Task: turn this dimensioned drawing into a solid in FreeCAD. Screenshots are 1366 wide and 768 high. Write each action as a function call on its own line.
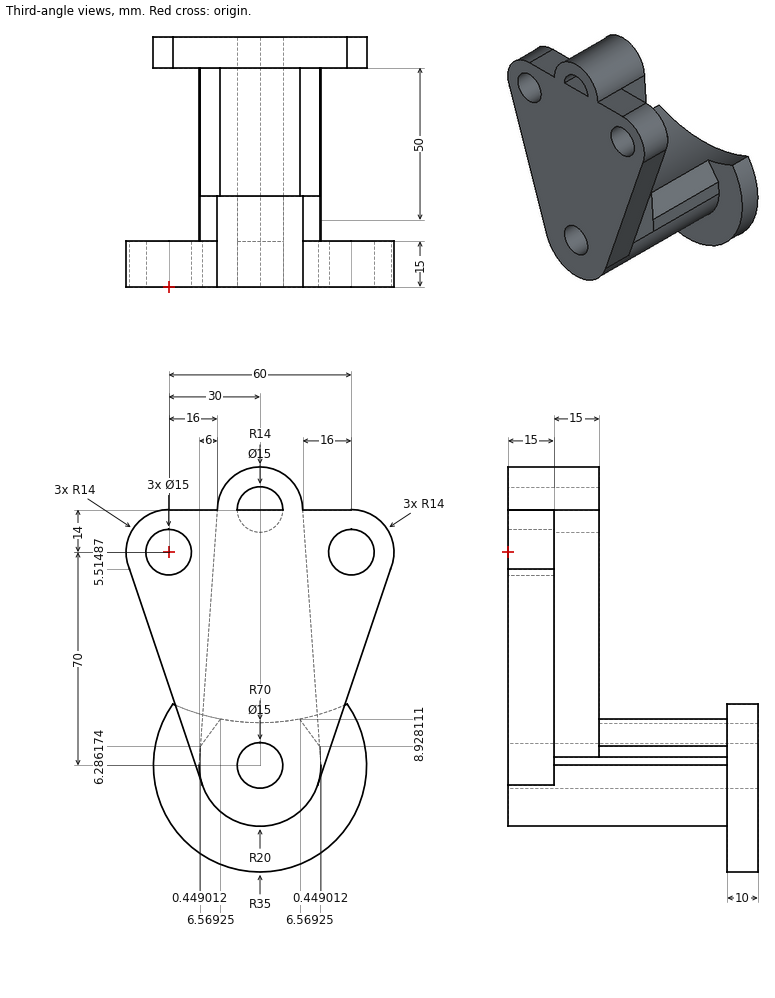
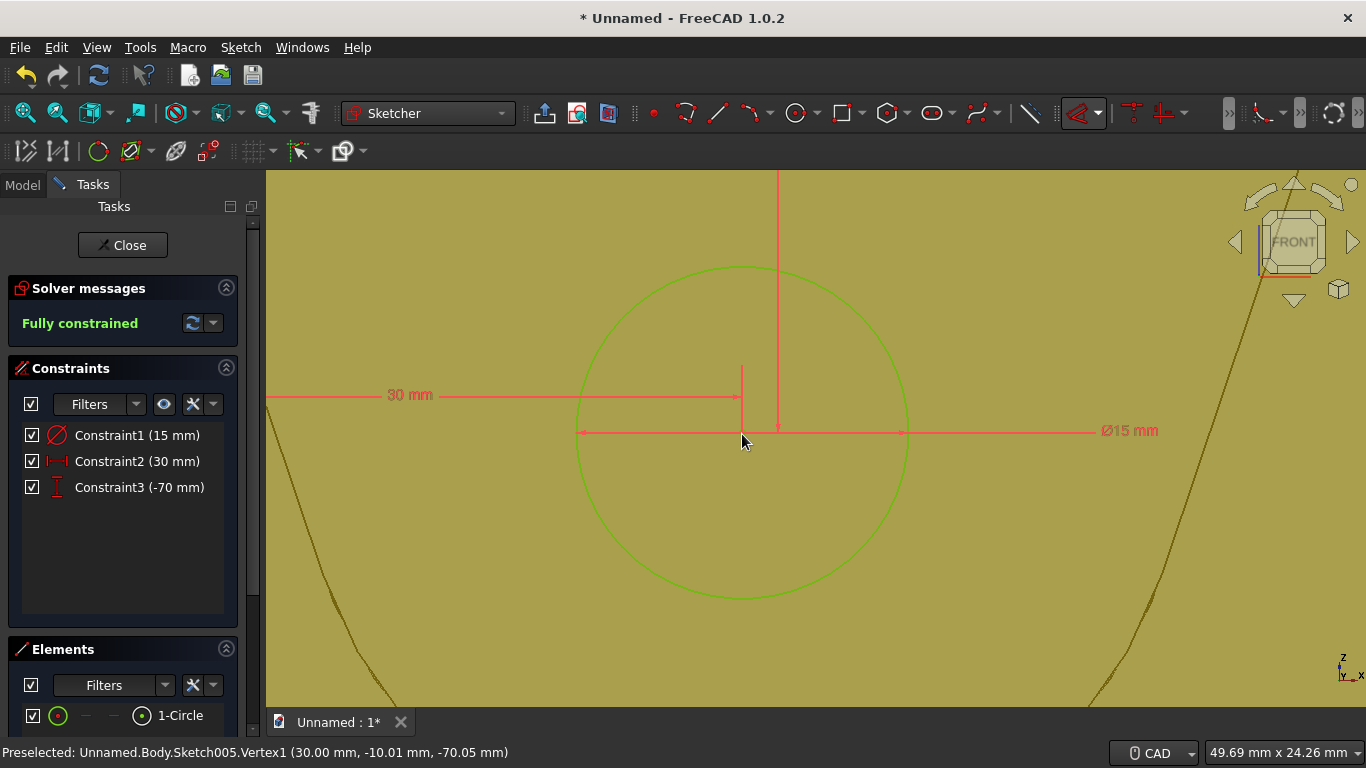
click(123, 245)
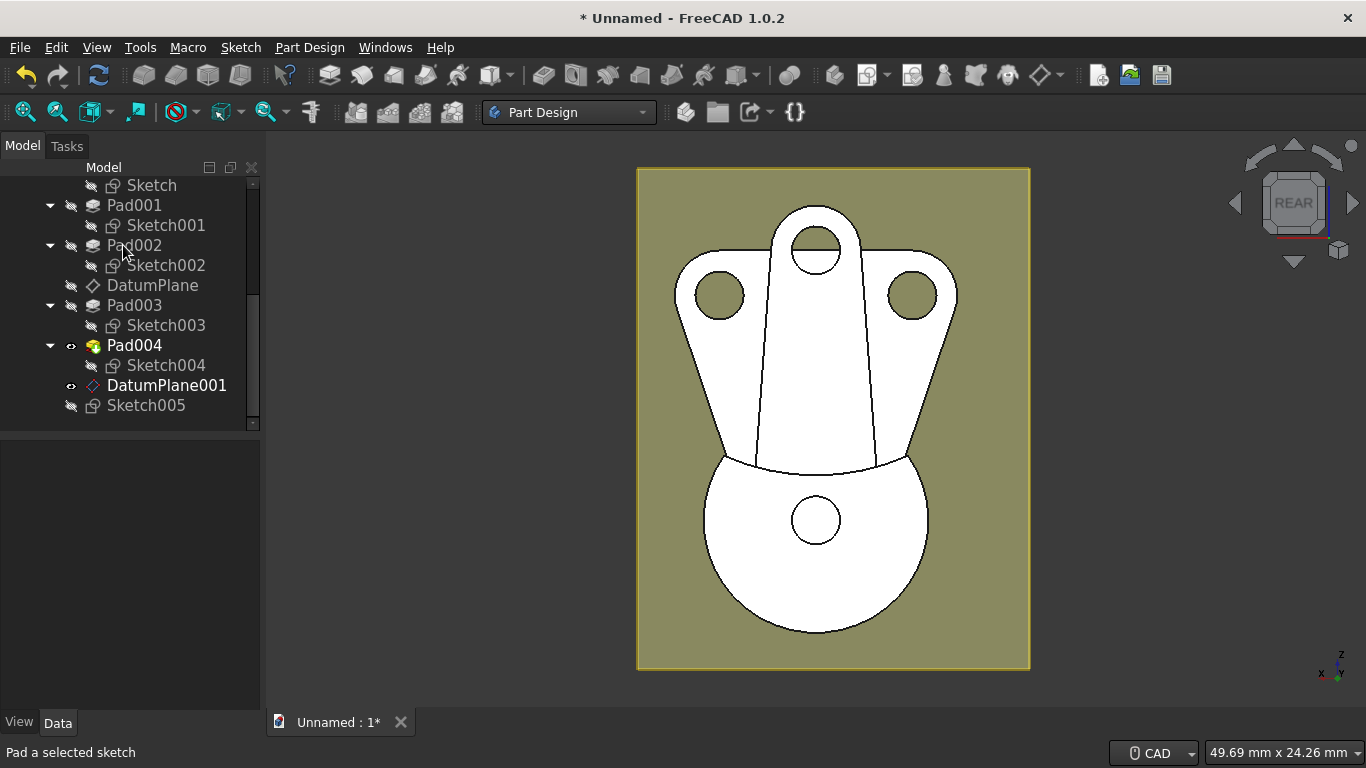
click(544, 76)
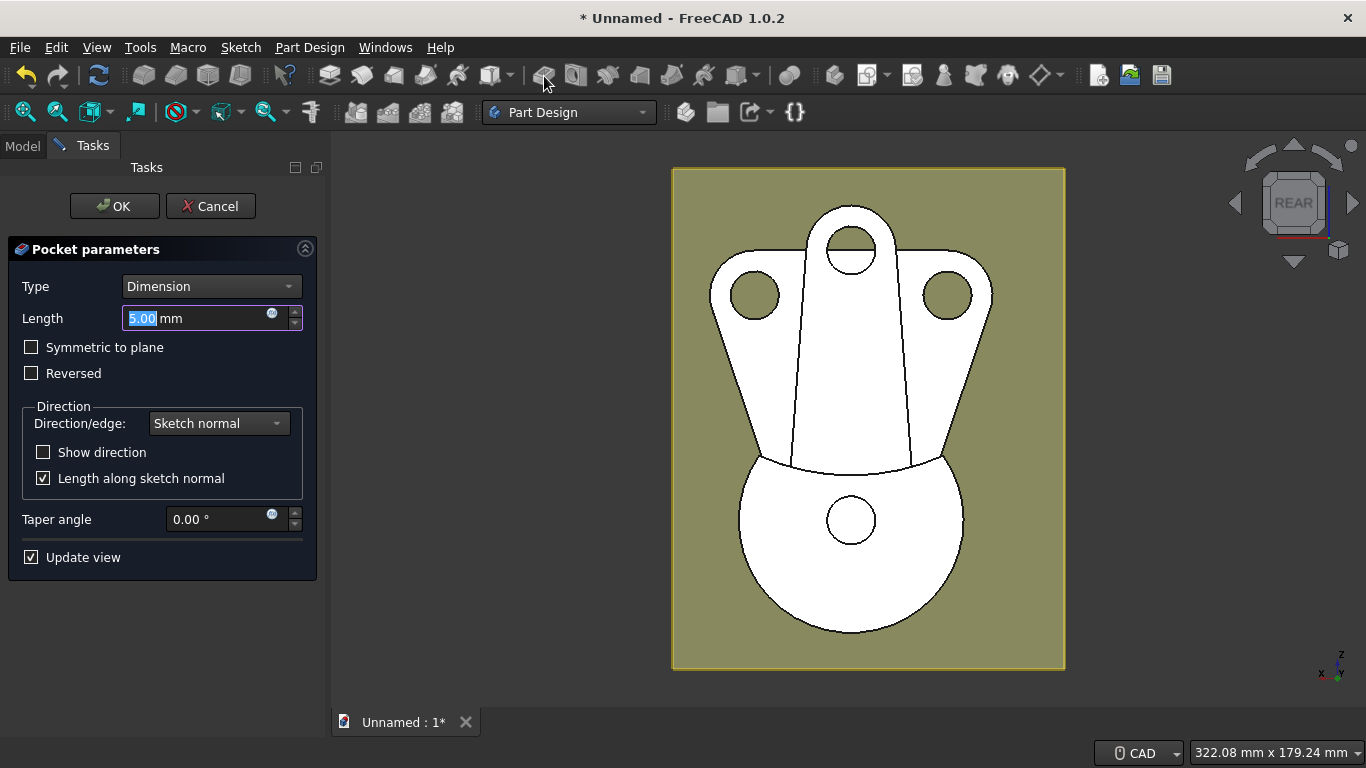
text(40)
key(Tab)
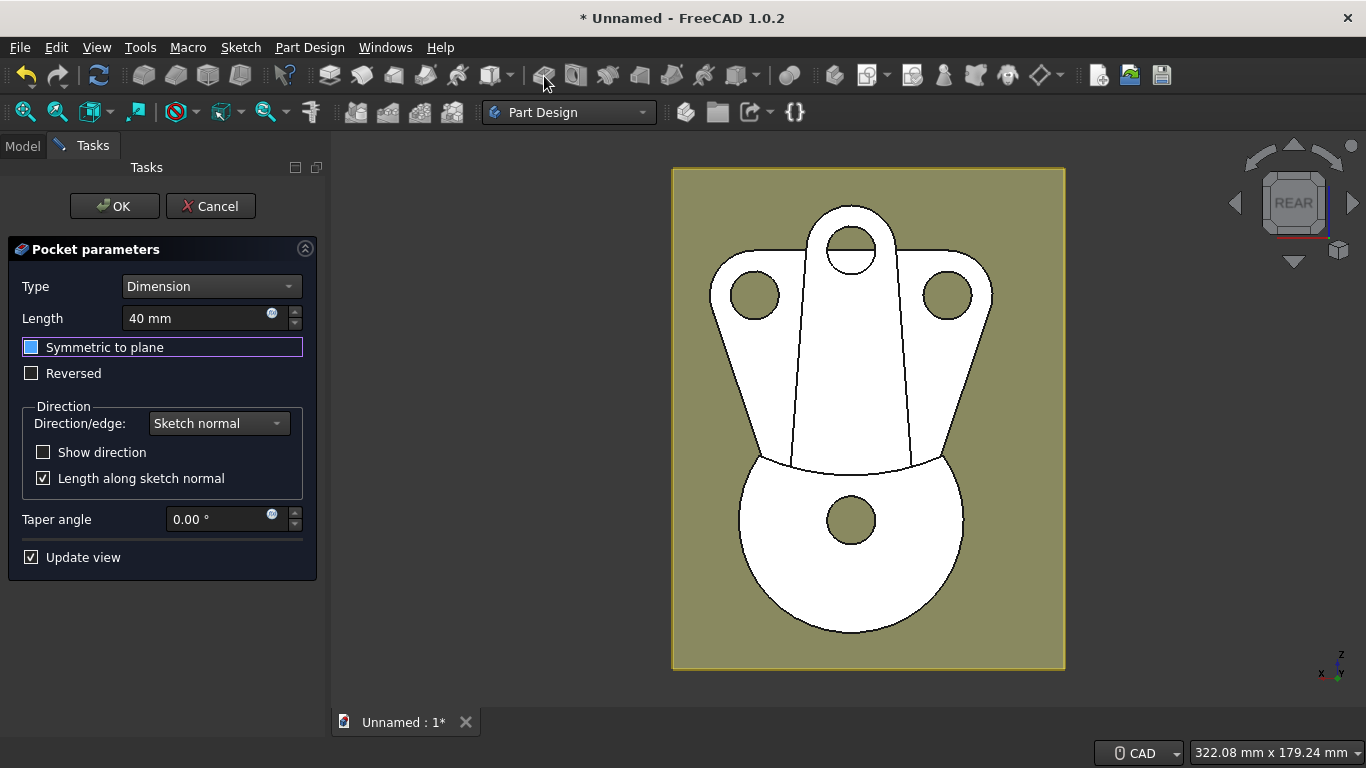
click(115, 206)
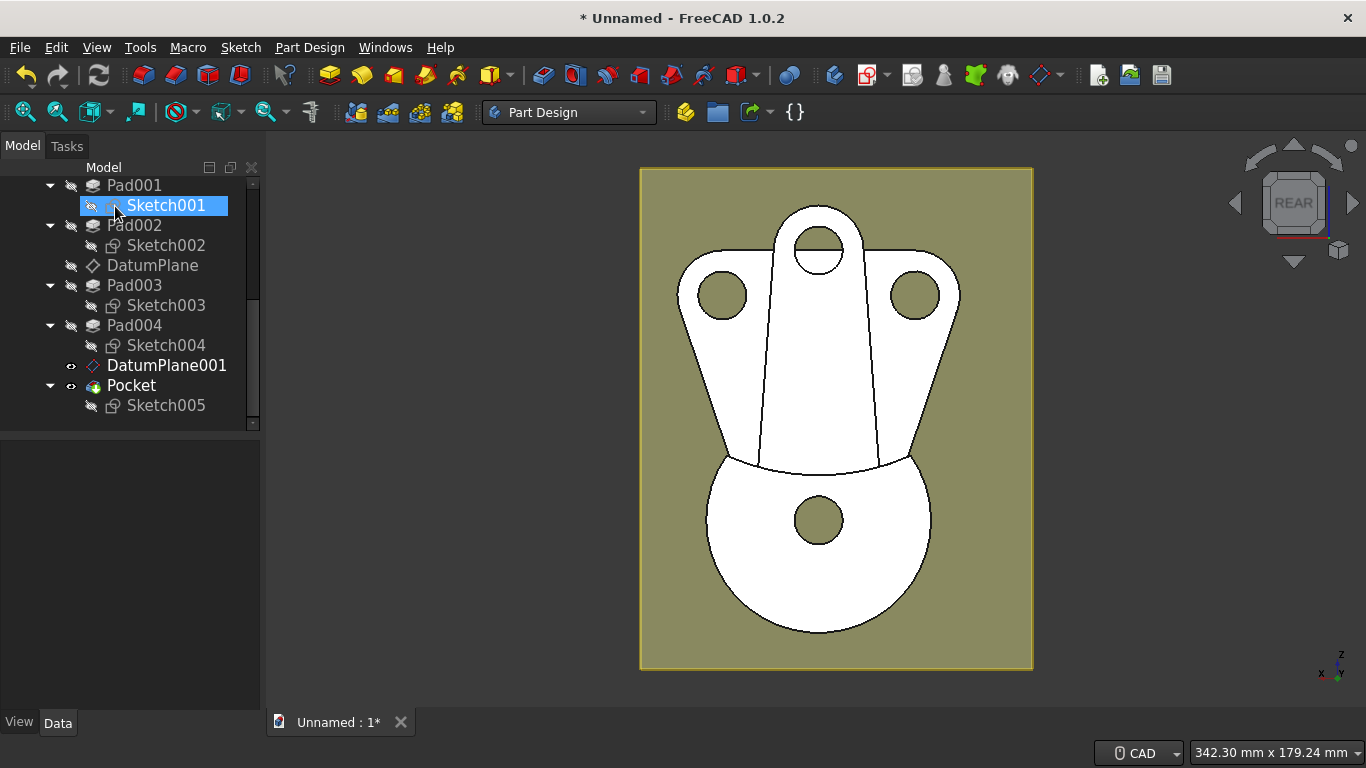
click(116, 366)
key(space)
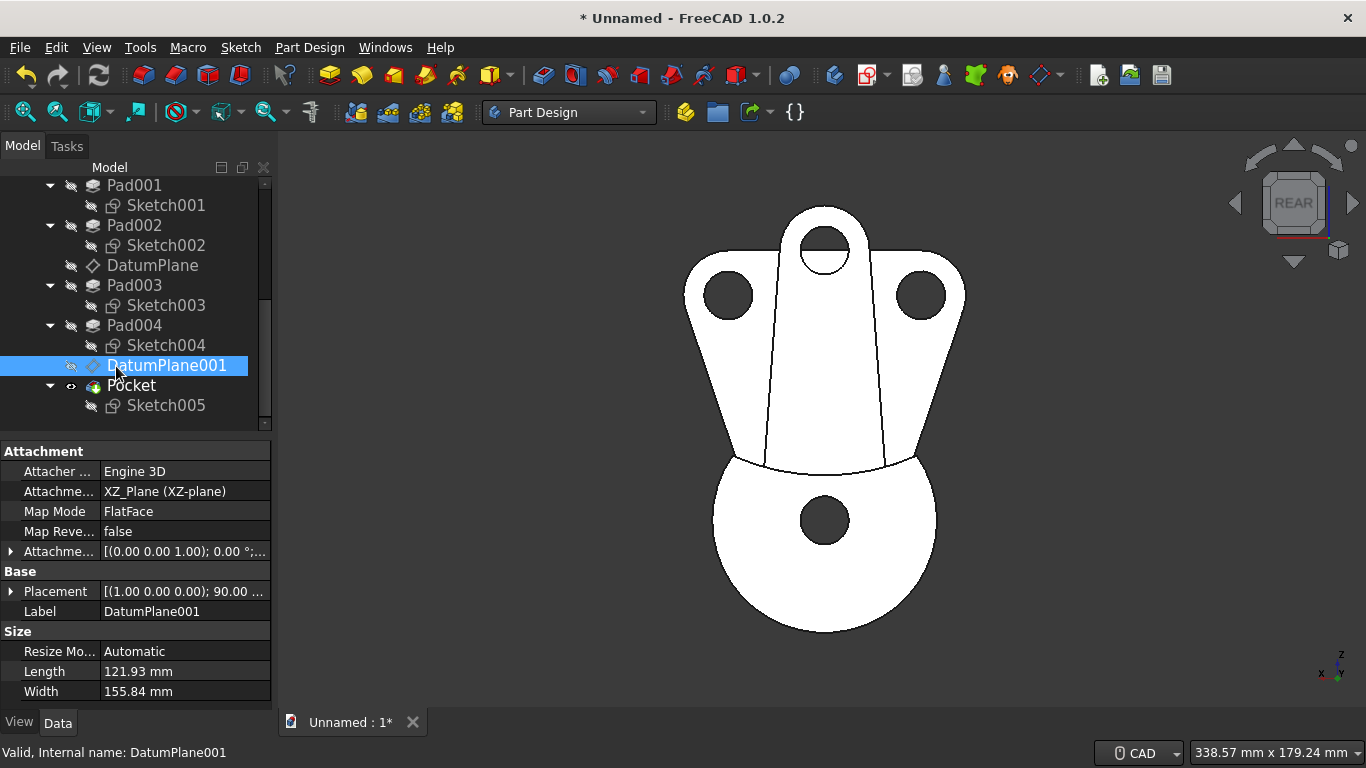
key(0)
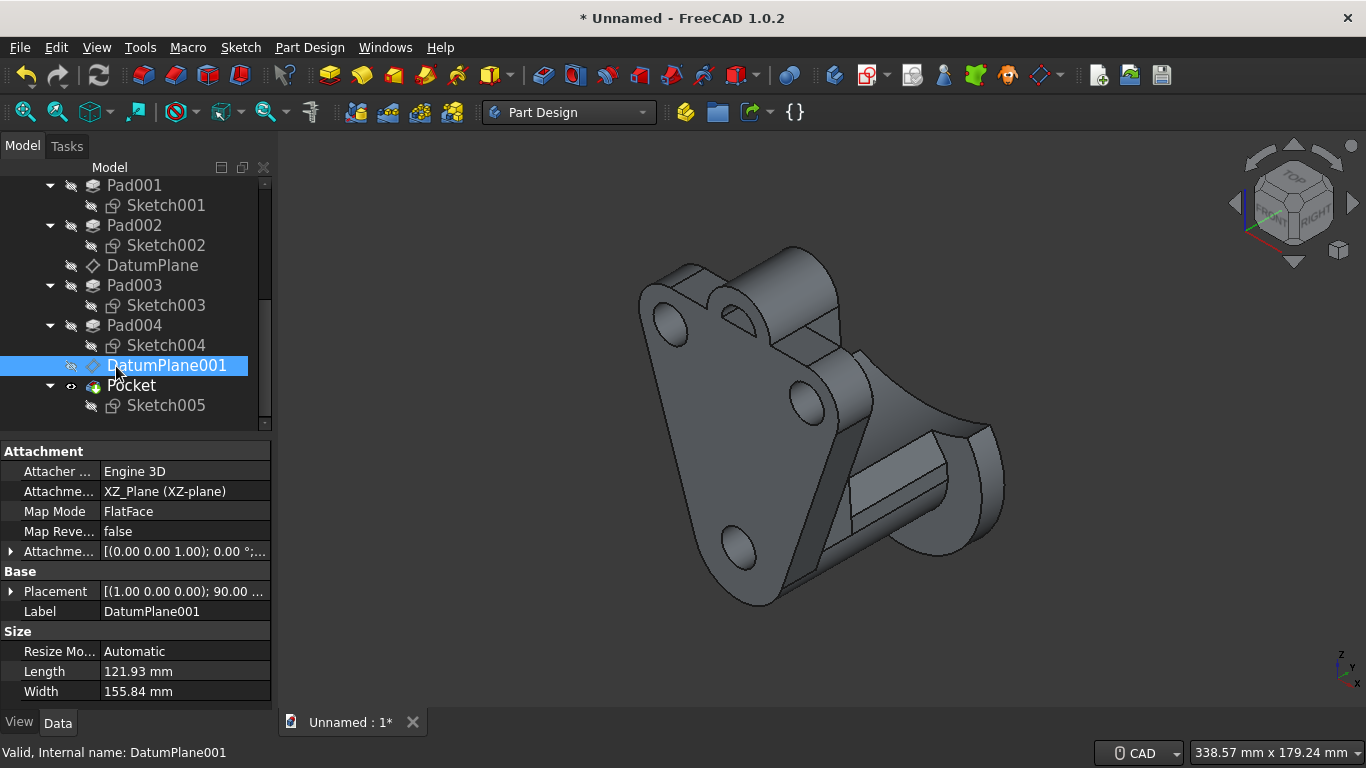
click(26, 112)